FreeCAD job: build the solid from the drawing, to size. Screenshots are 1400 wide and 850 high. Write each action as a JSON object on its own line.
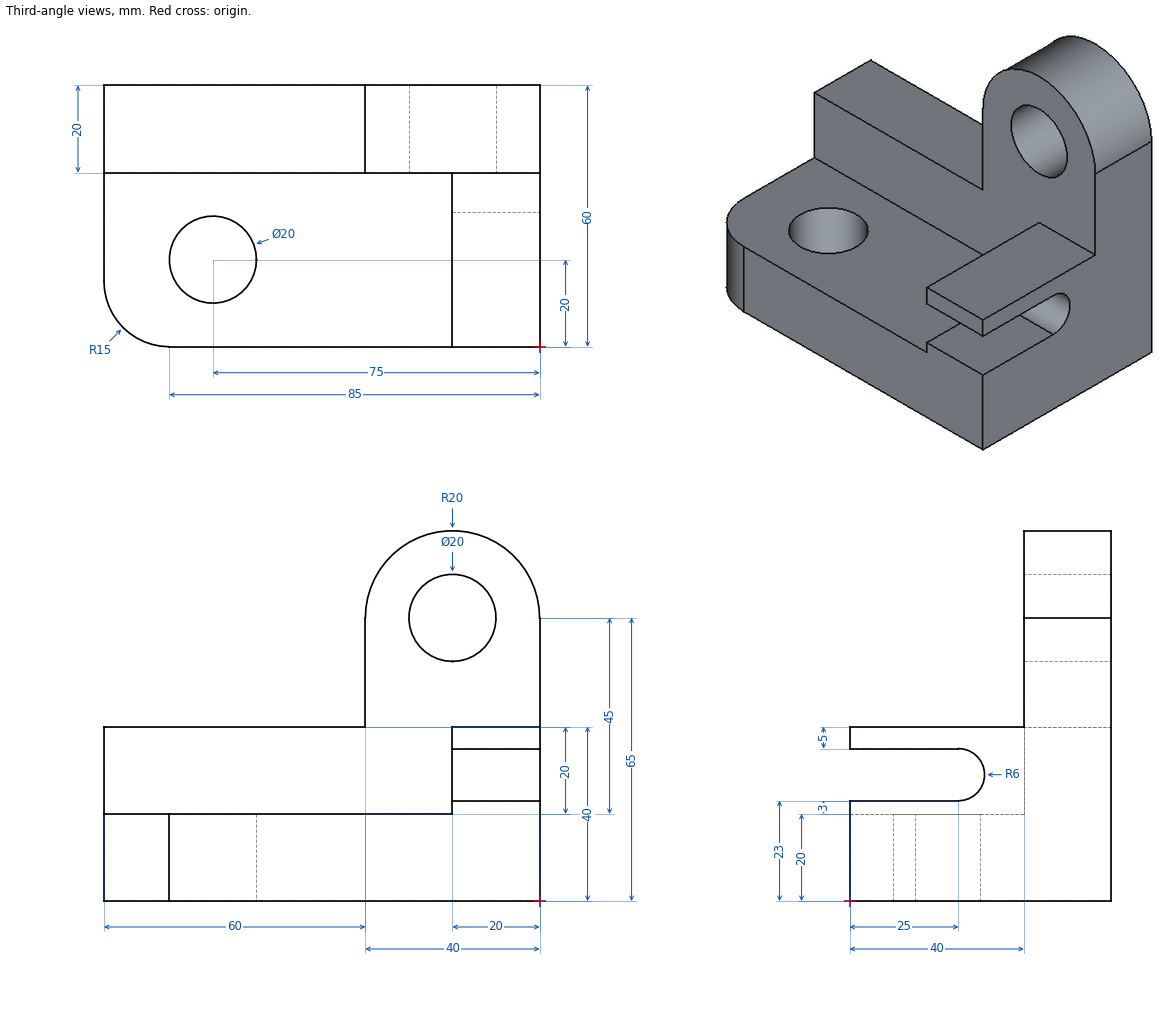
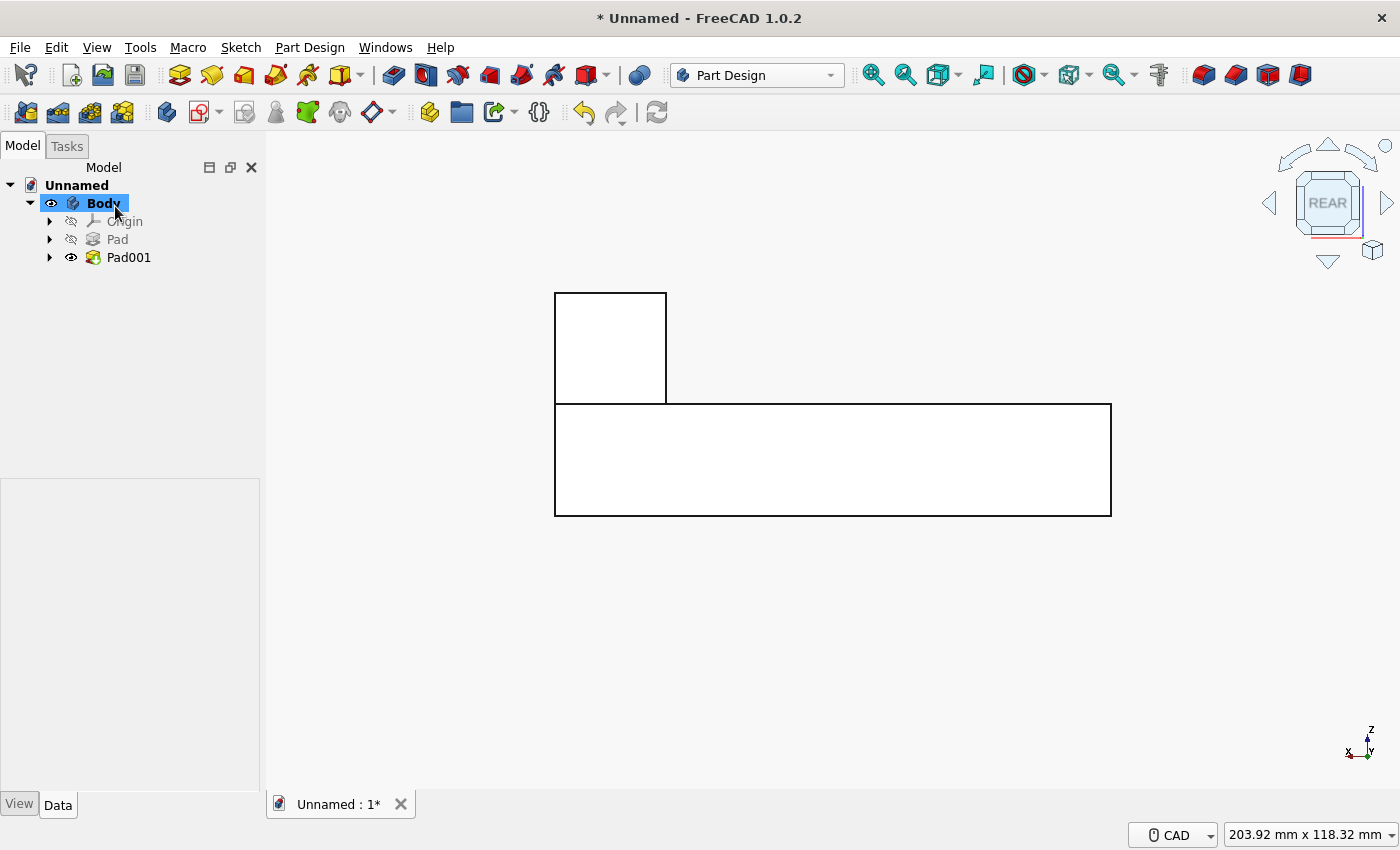
{"action": "left_click", "coordinate": [674, 459]}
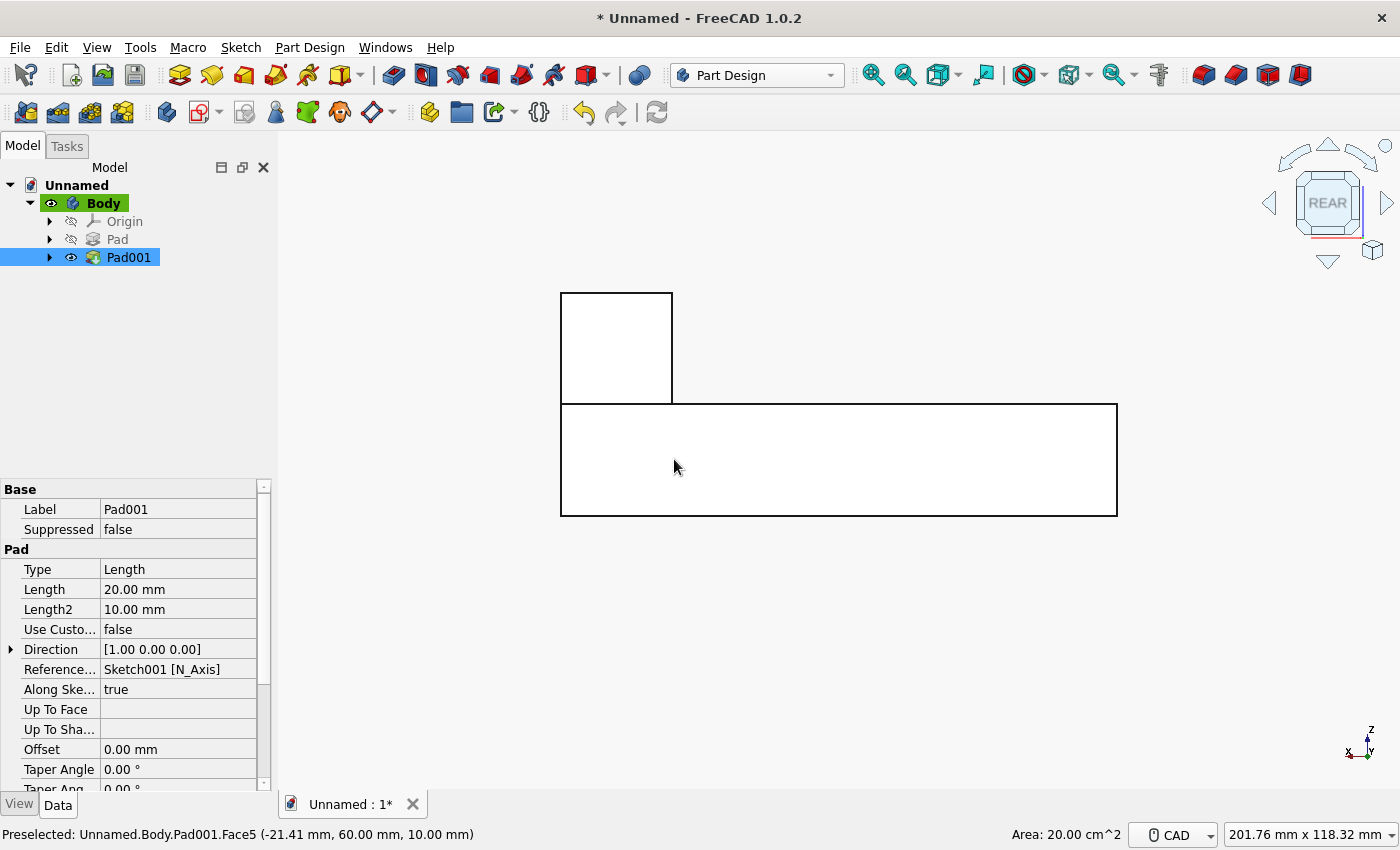
{"action": "left_click", "coordinate": [200, 112]}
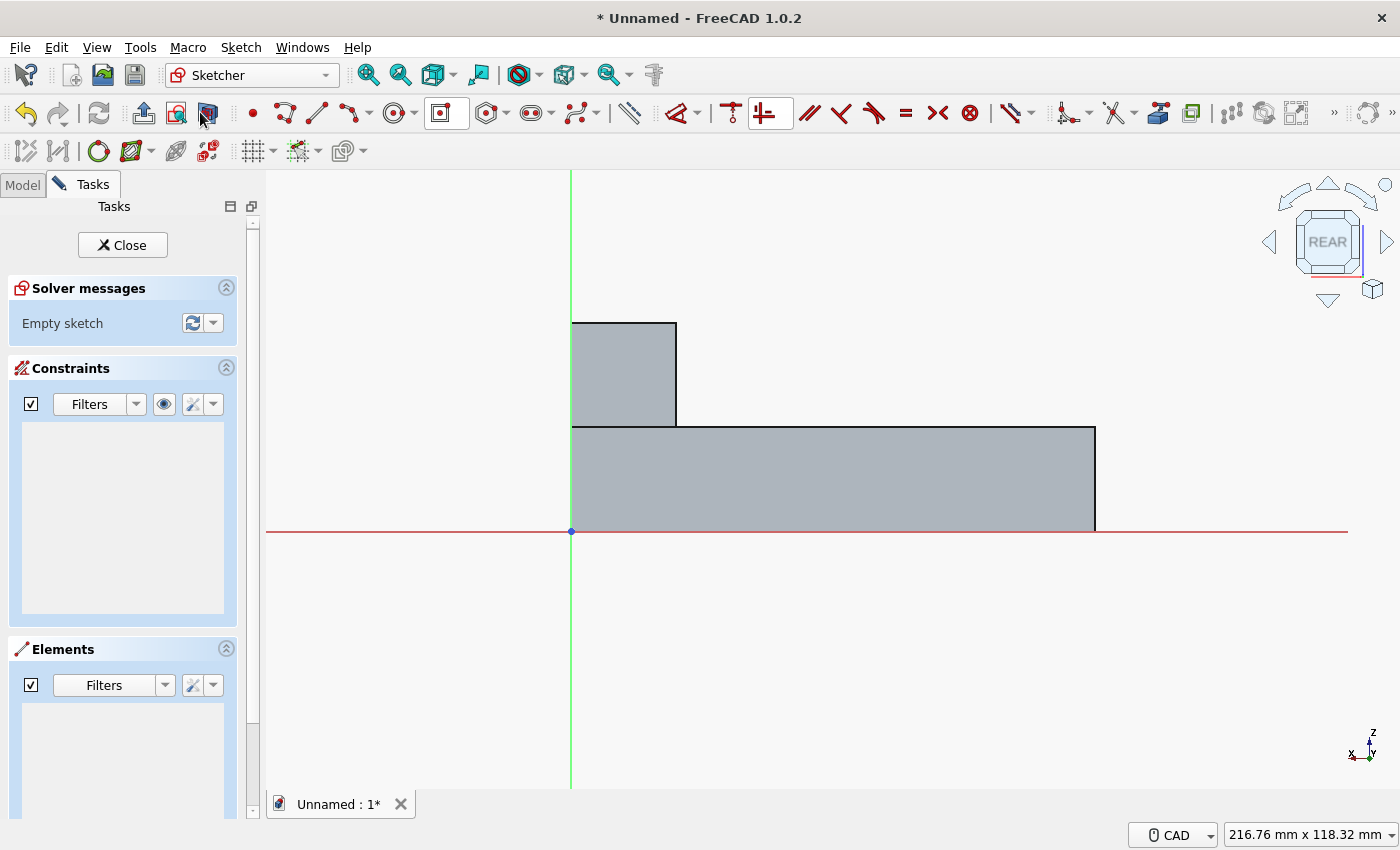
{"action": "key", "text": "g r"}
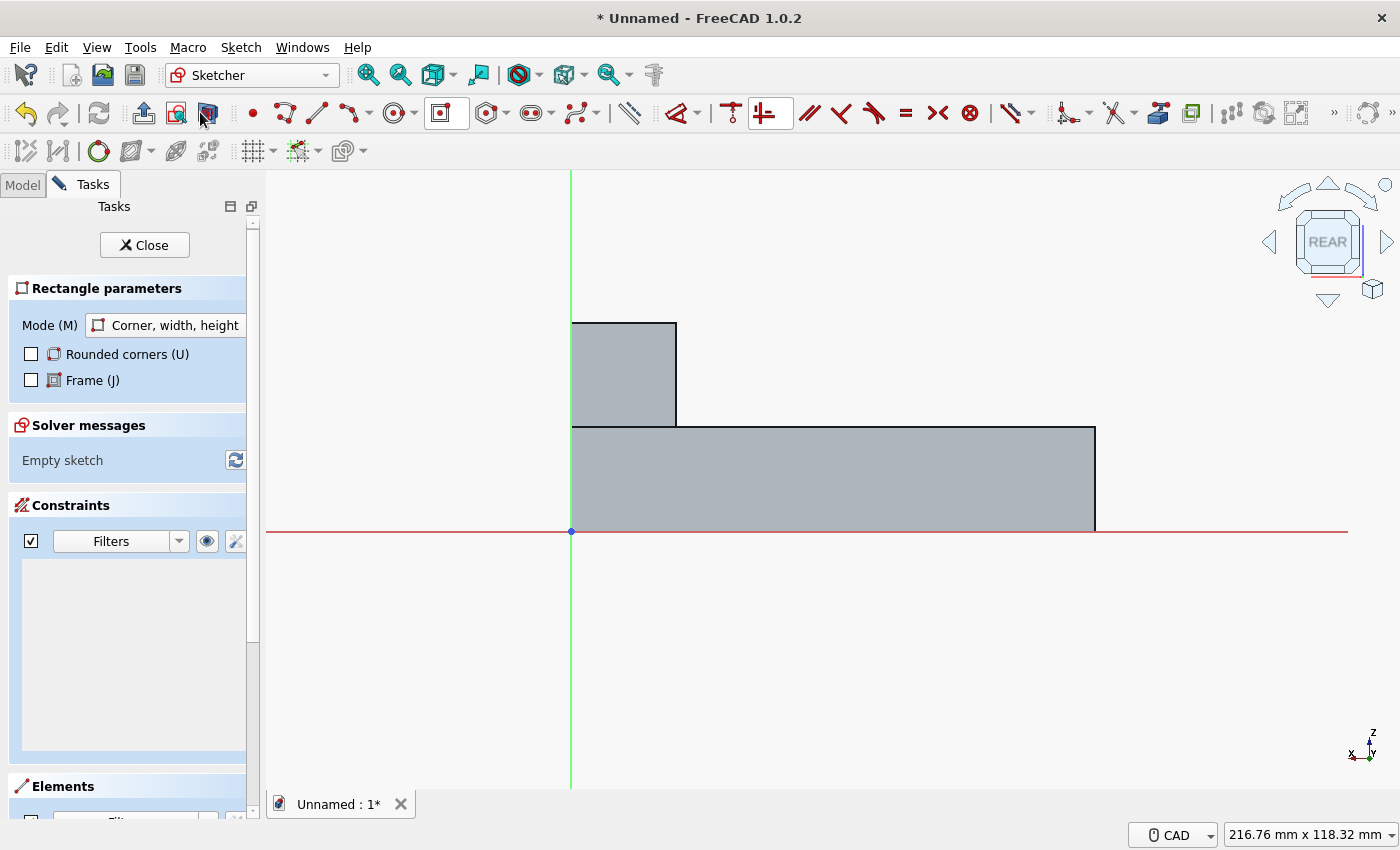
{"action": "left_click", "coordinate": [781, 323]}
{"action": "left_click", "coordinate": [1095, 427]}
{"action": "key", "text": "Escape"}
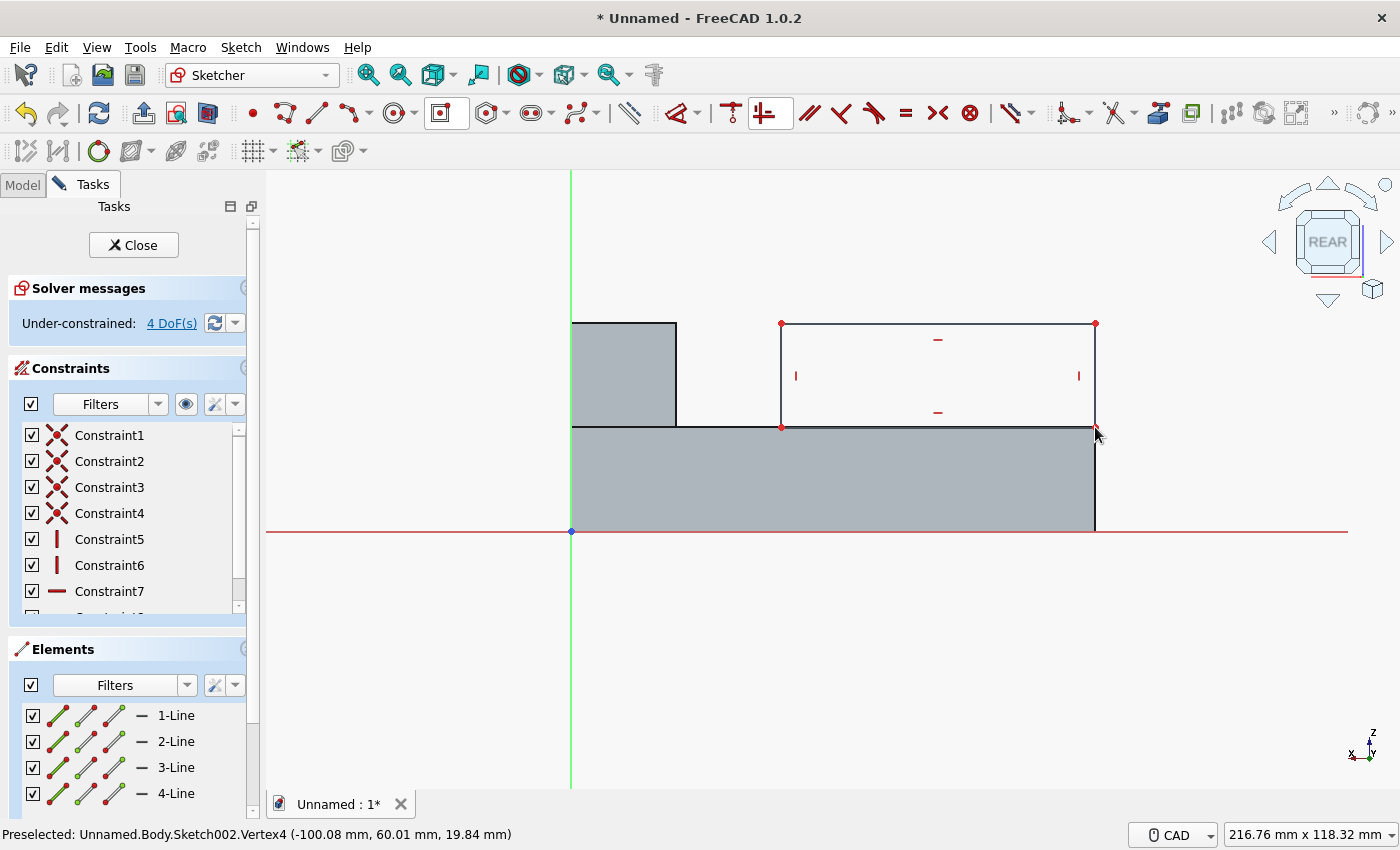
{"action": "left_click", "coordinate": [676, 114]}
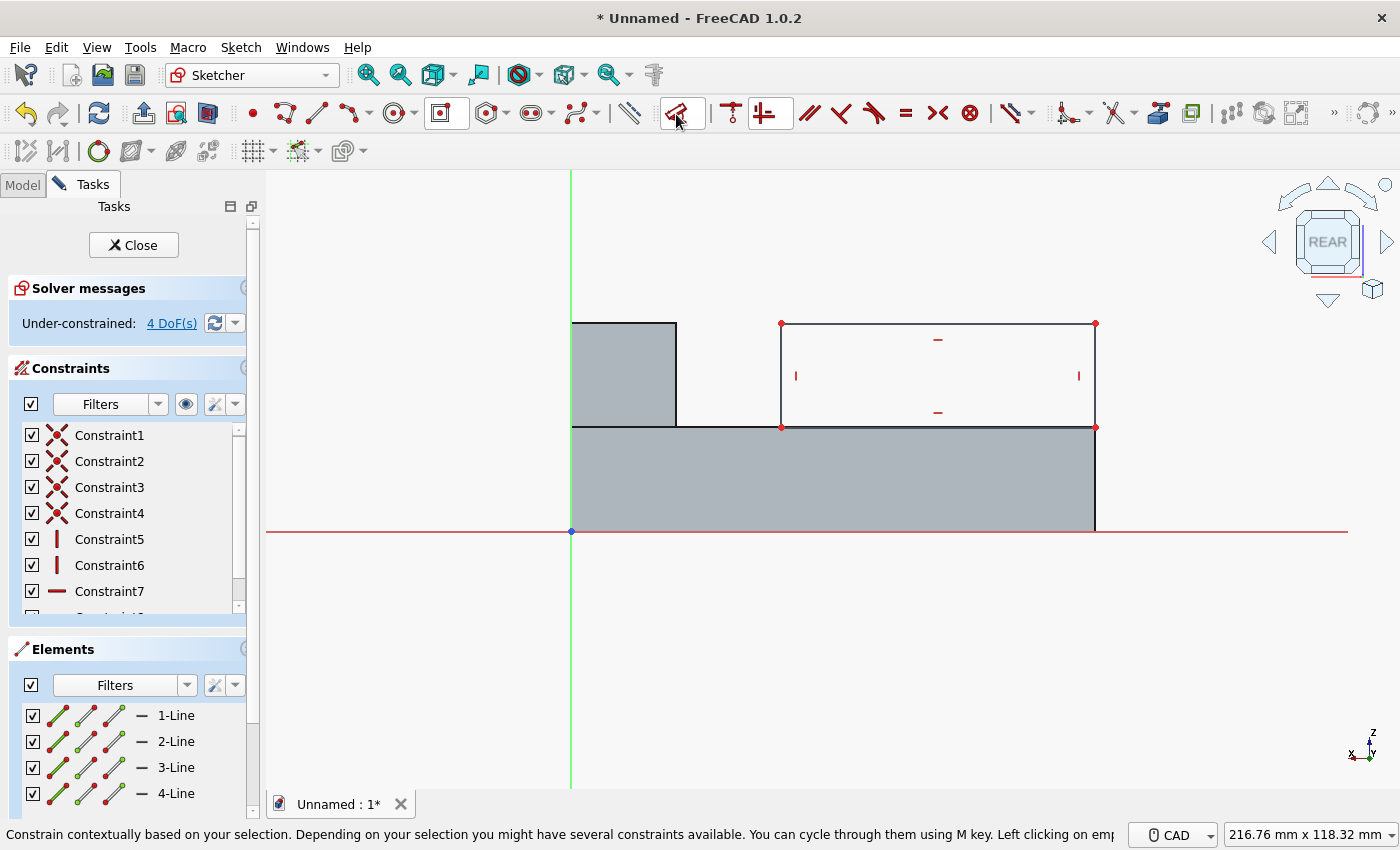
{"action": "left_click", "coordinate": [781, 355]}
{"action": "left_click", "coordinate": [747, 376]}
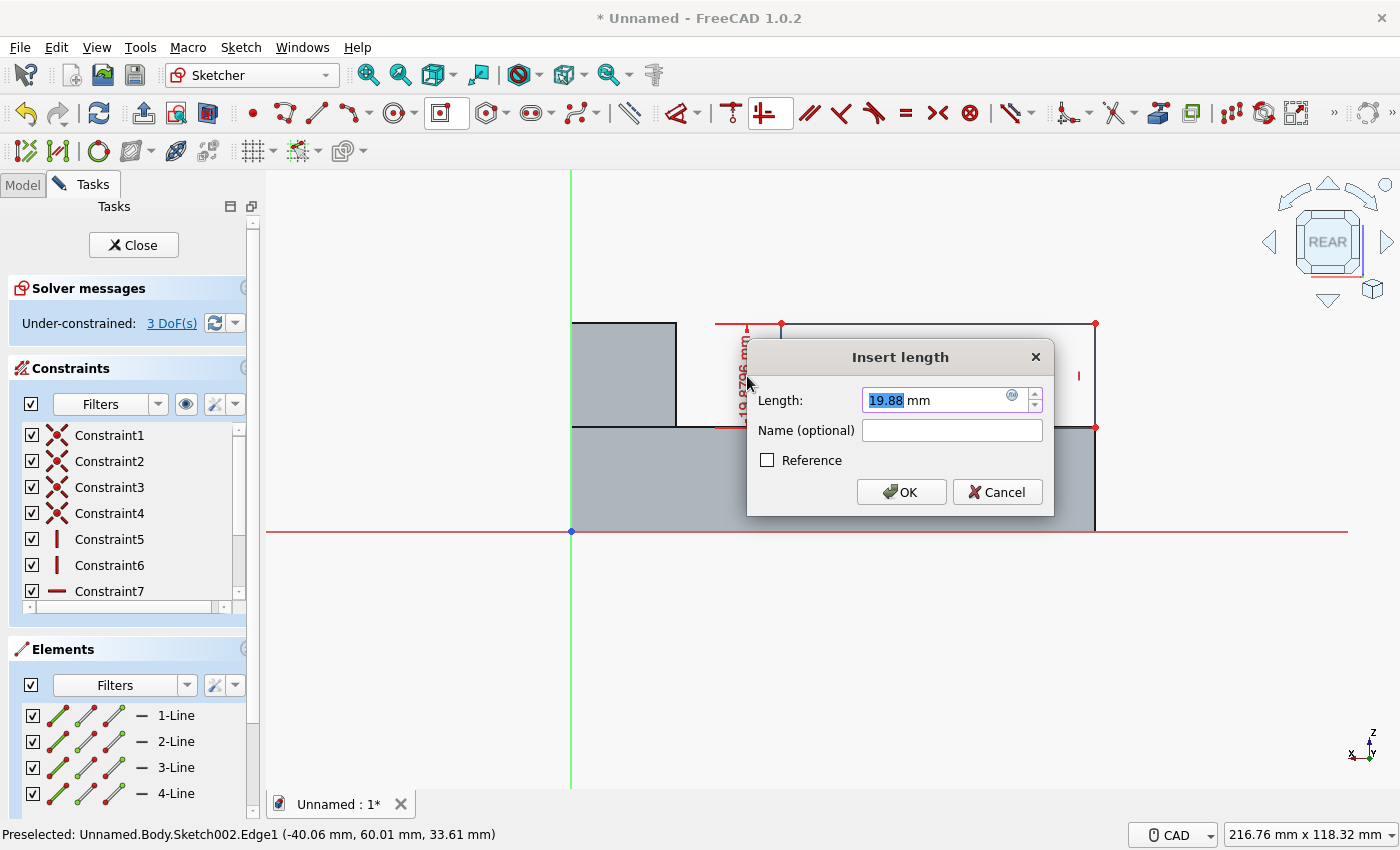
{"action": "type", "text": "20"}
{"action": "key", "text": "Return"}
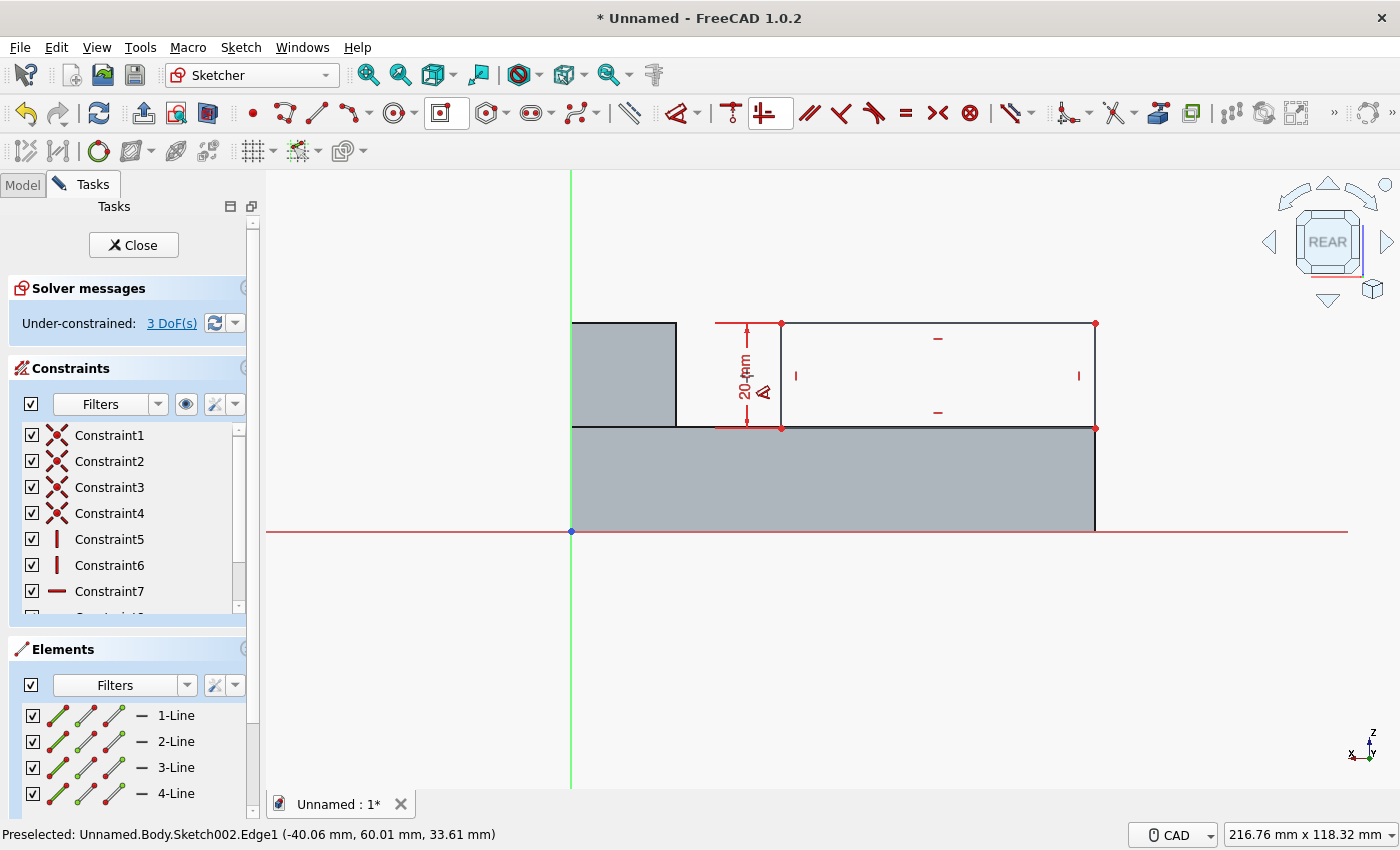
{"action": "left_click", "coordinate": [875, 428]}
{"action": "left_click", "coordinate": [938, 462]}